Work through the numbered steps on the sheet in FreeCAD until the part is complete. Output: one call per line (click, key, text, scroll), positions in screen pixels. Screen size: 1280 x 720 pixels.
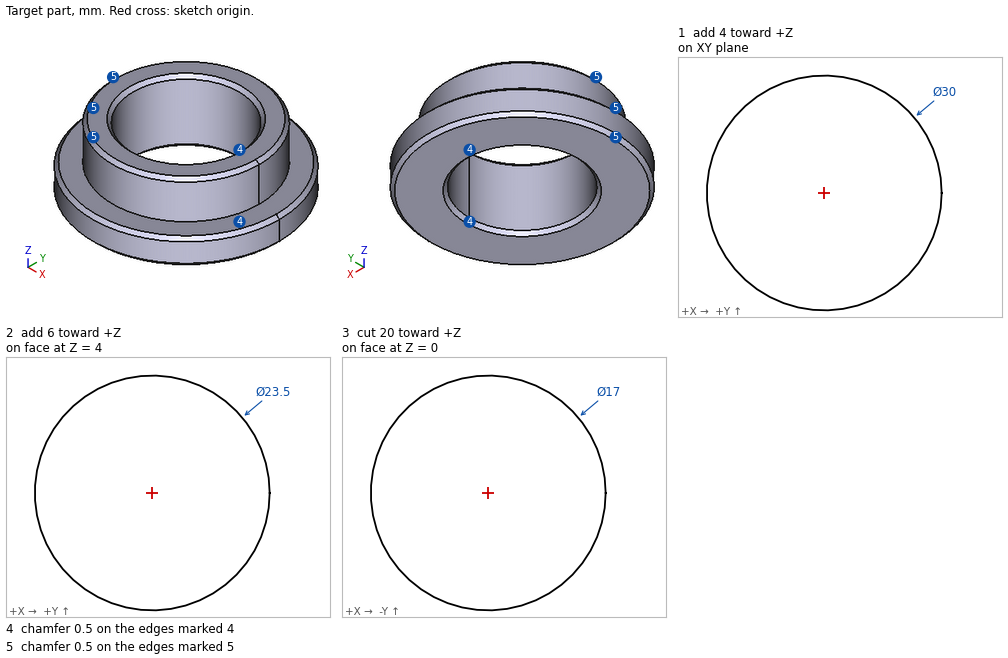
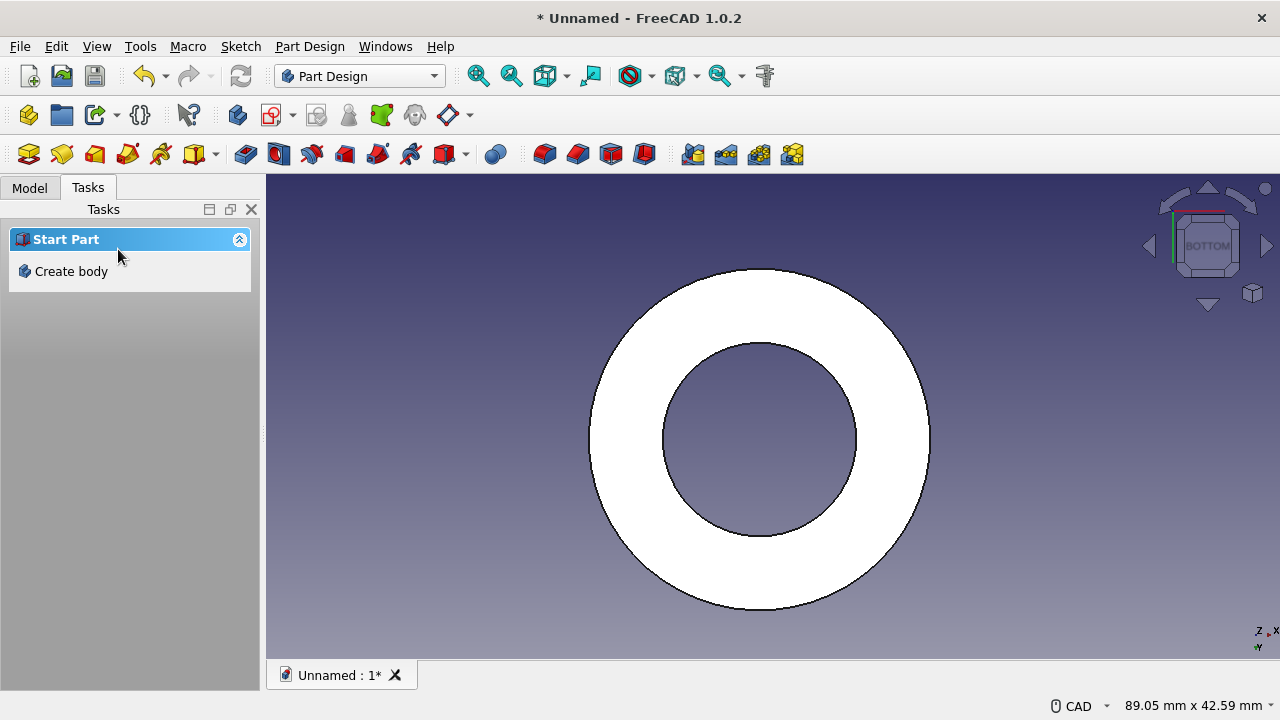
click(663, 439)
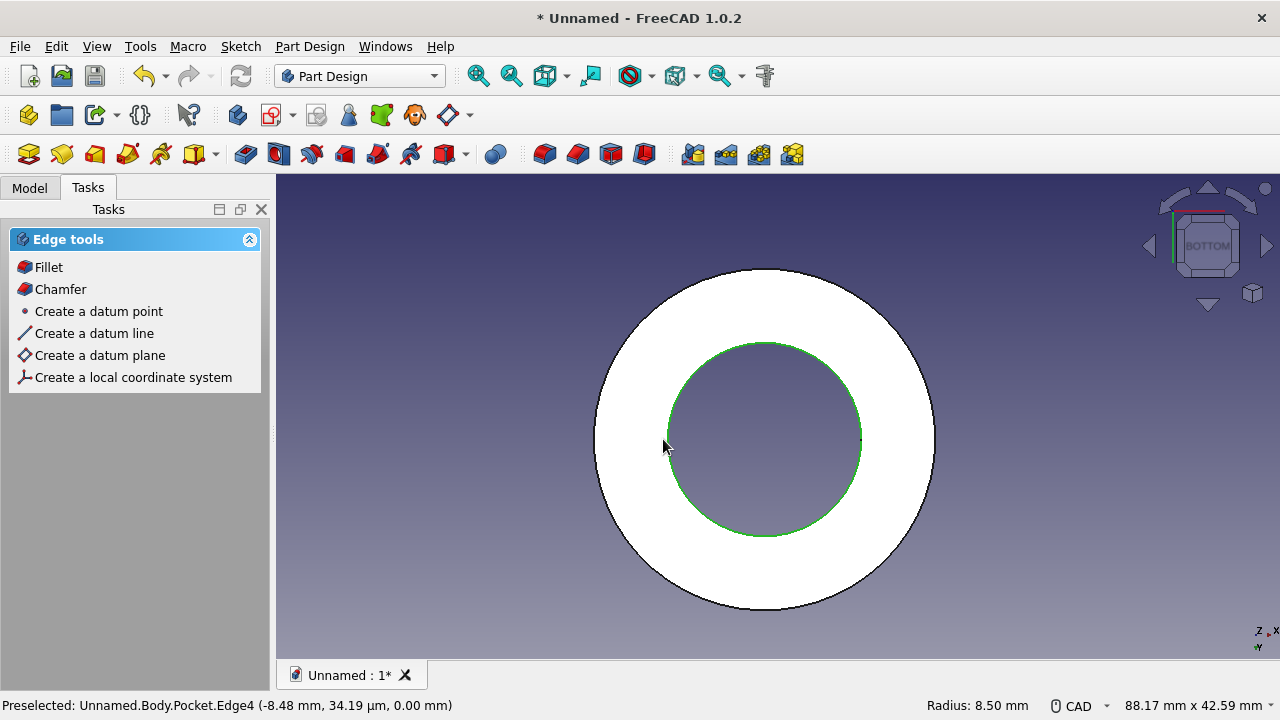
key(0)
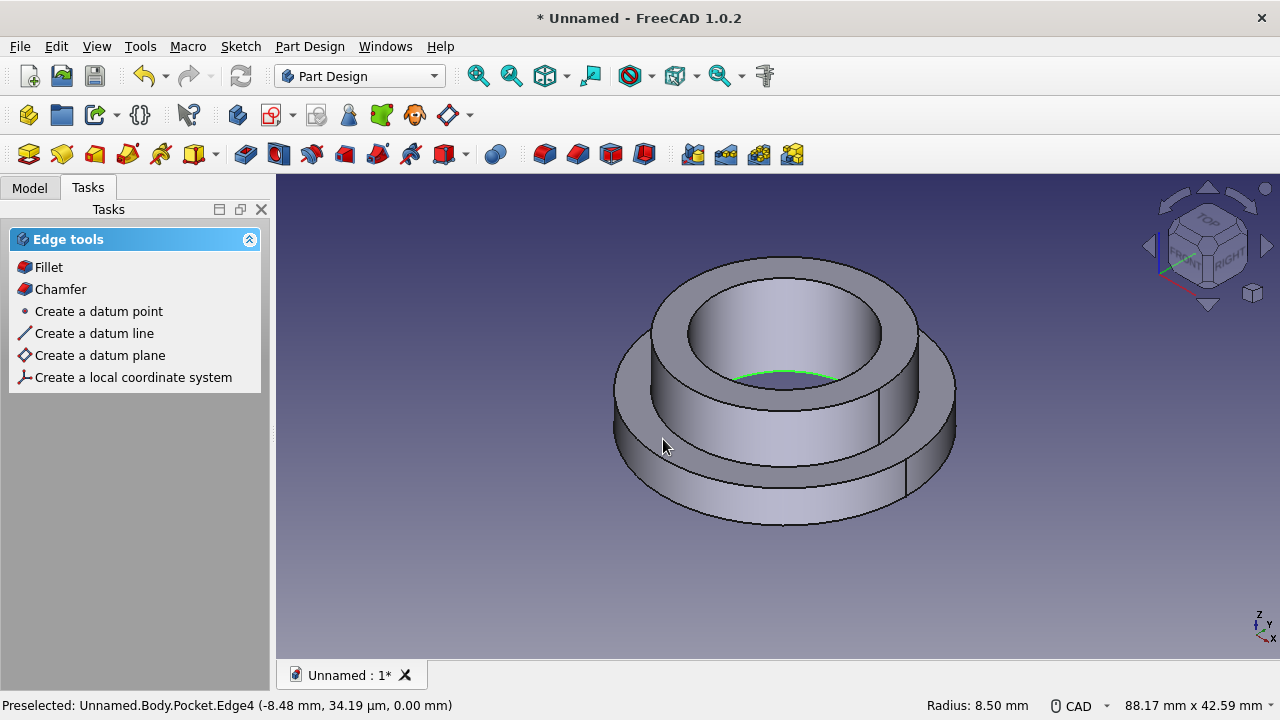
click(716, 293, ctrl)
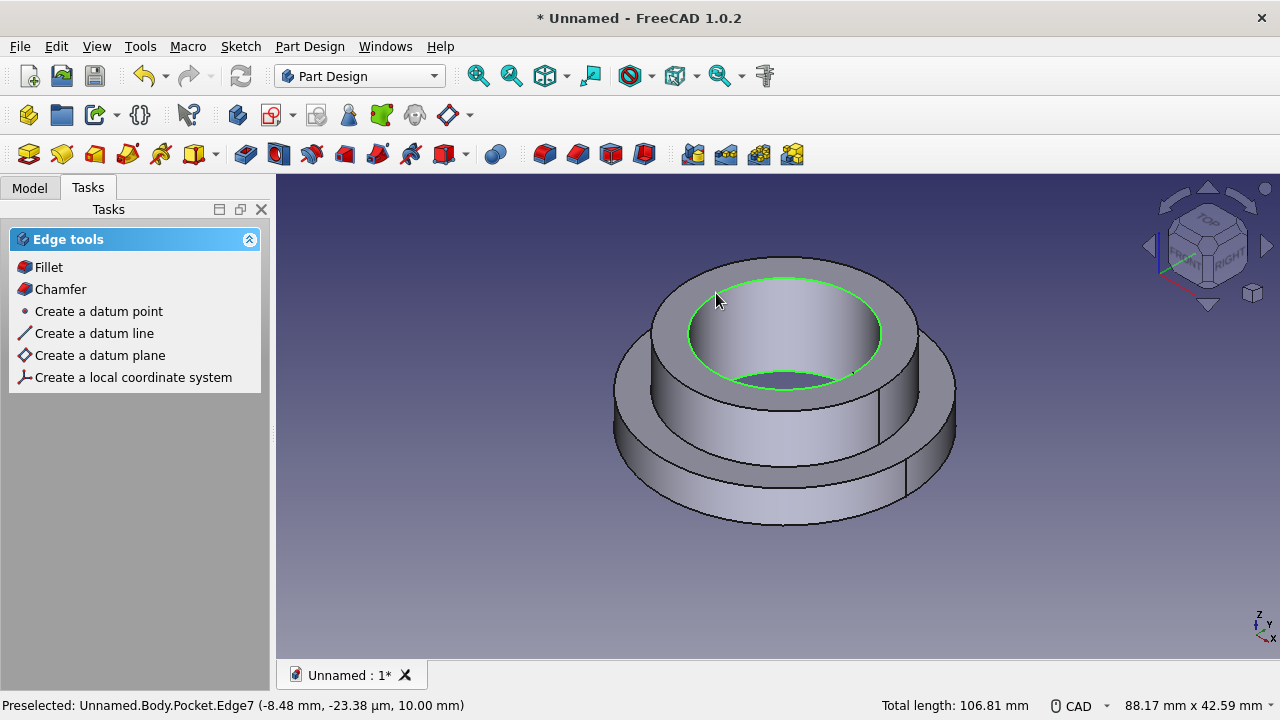
click(578, 154)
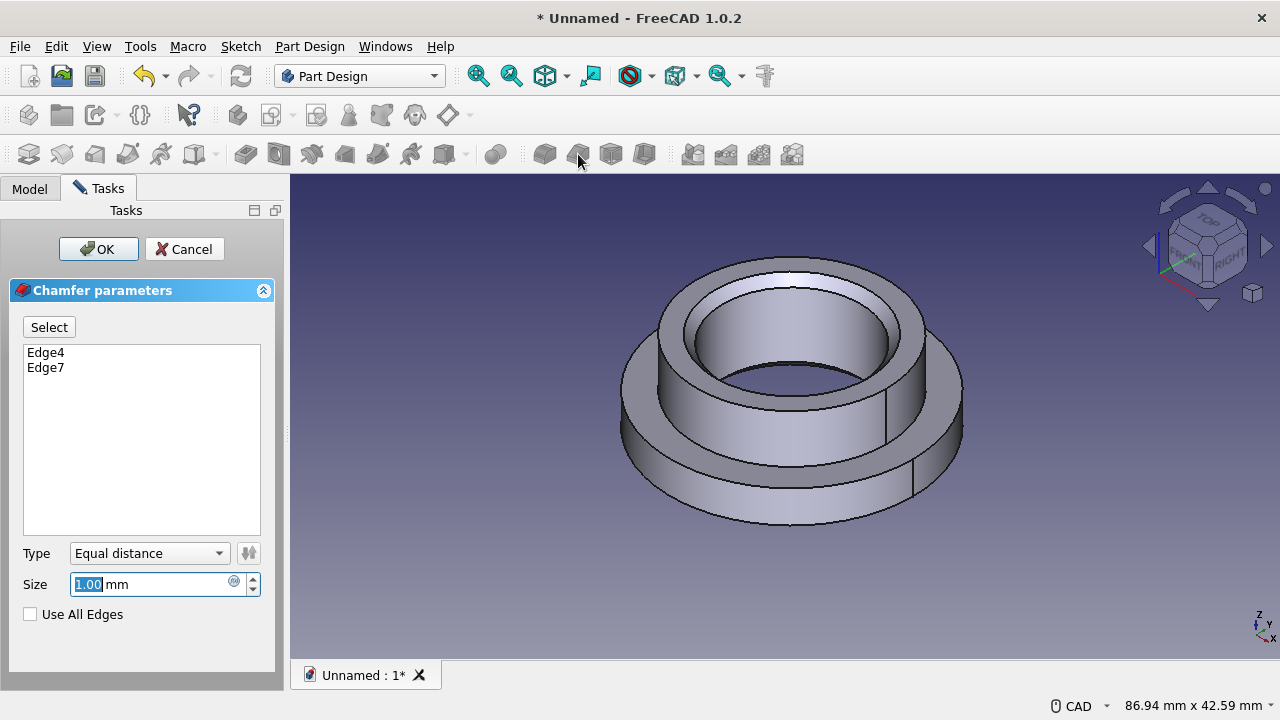
text(0.5)
key(Tab)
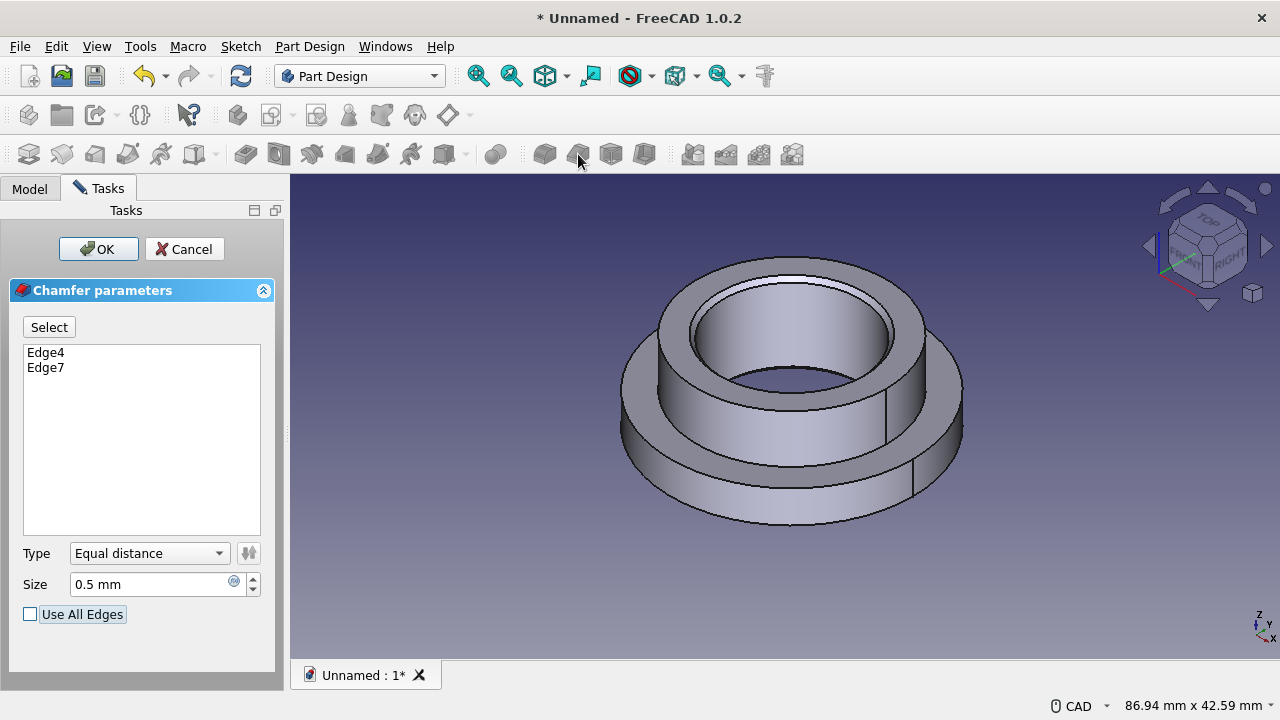
click(99, 249)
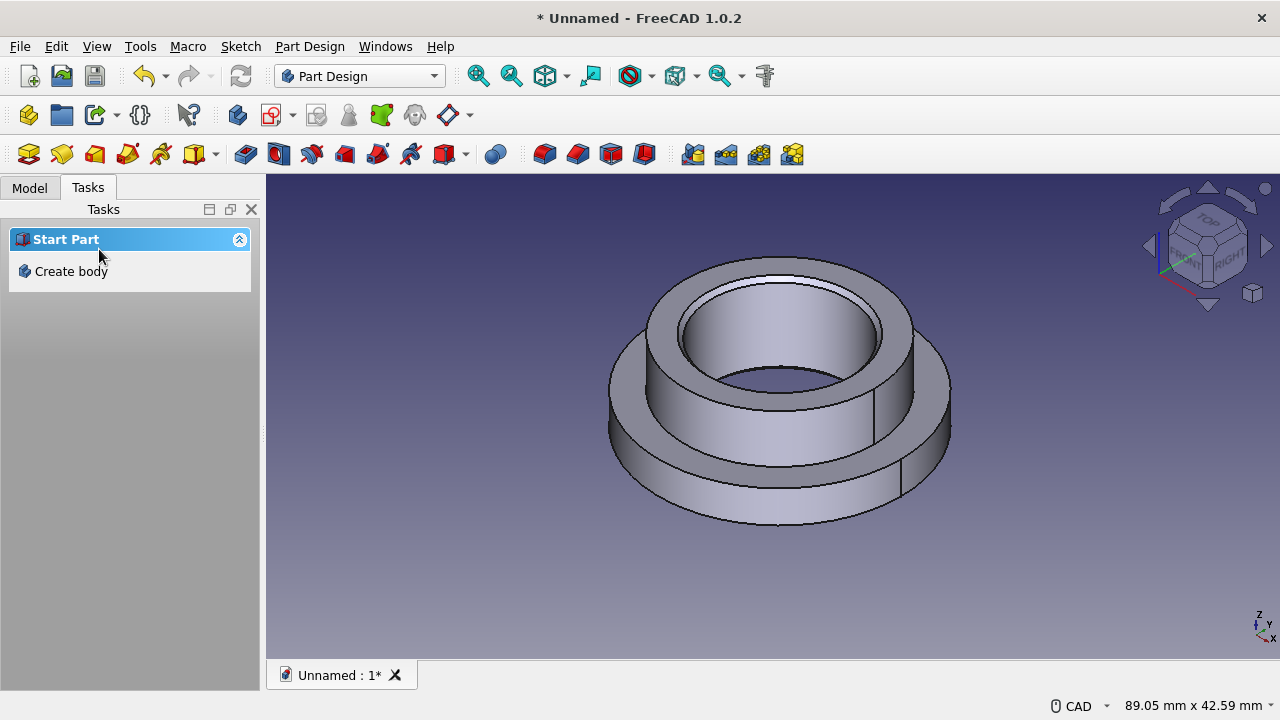
click(628, 434)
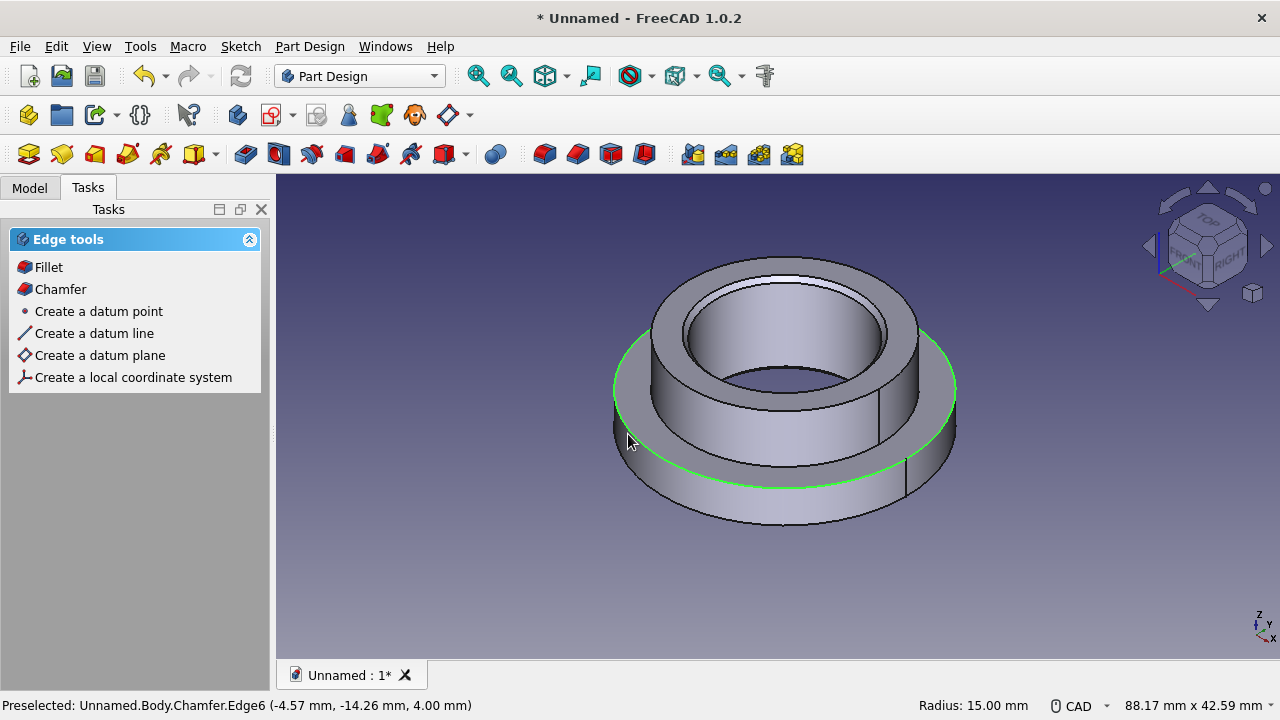
click(666, 368, ctrl)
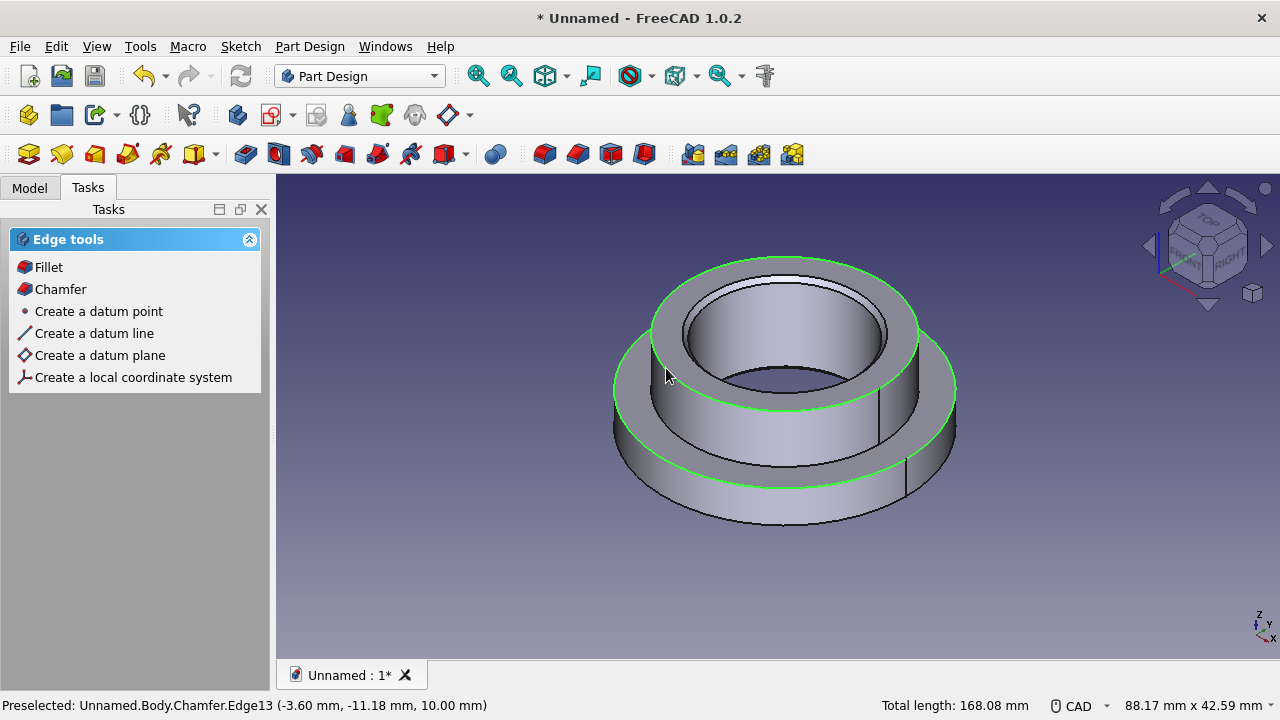
key(2)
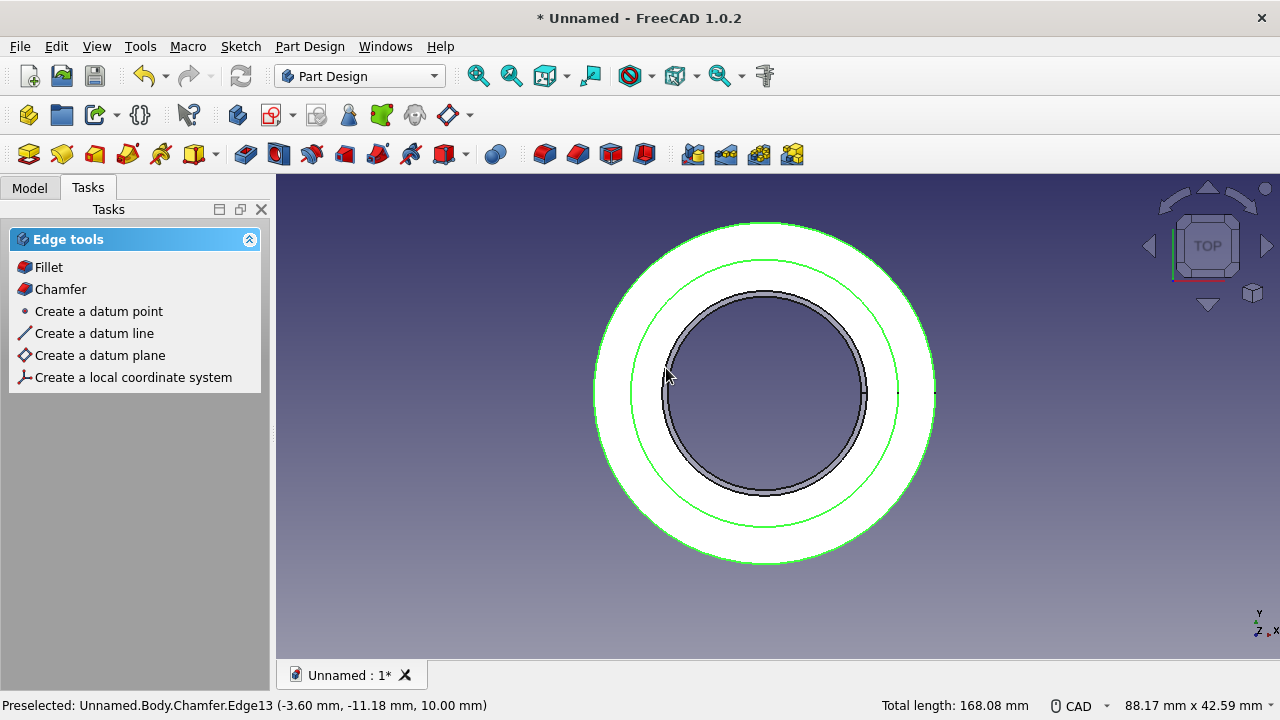
key(0)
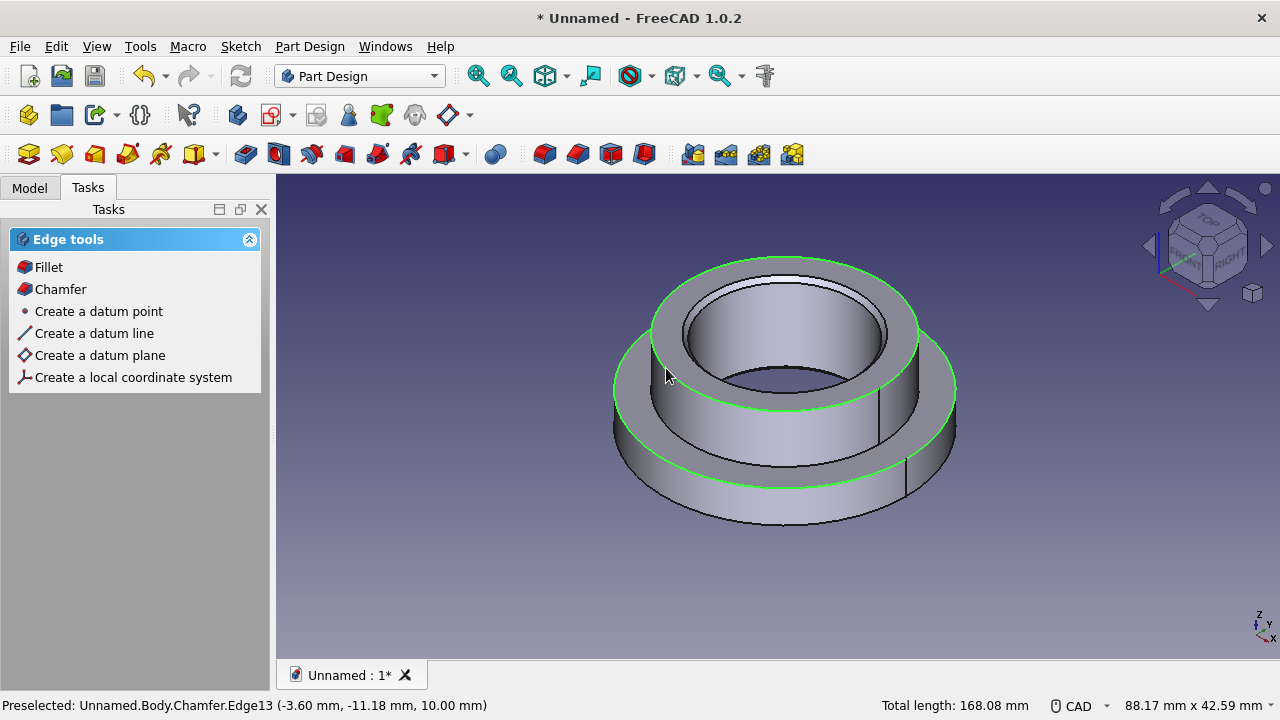
key(1)